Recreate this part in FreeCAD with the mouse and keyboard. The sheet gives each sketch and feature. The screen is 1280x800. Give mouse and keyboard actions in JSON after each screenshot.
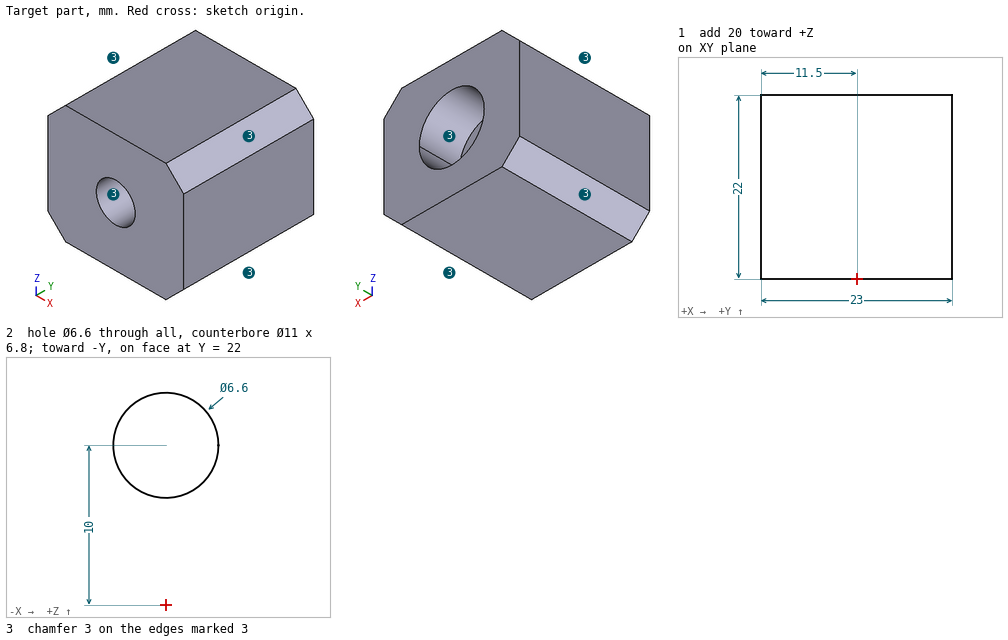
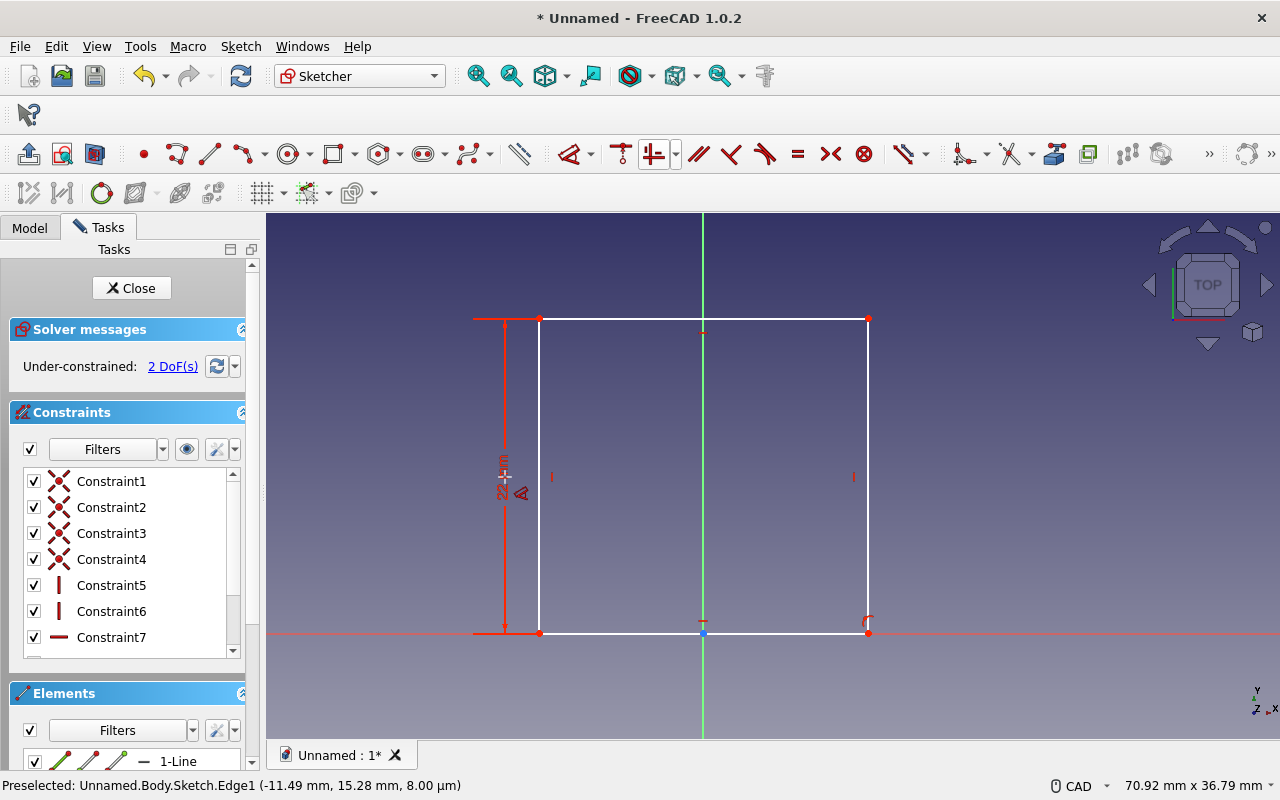
{"action": "left_click", "coordinate": [638, 634]}
{"action": "left_click", "coordinate": [628, 668]}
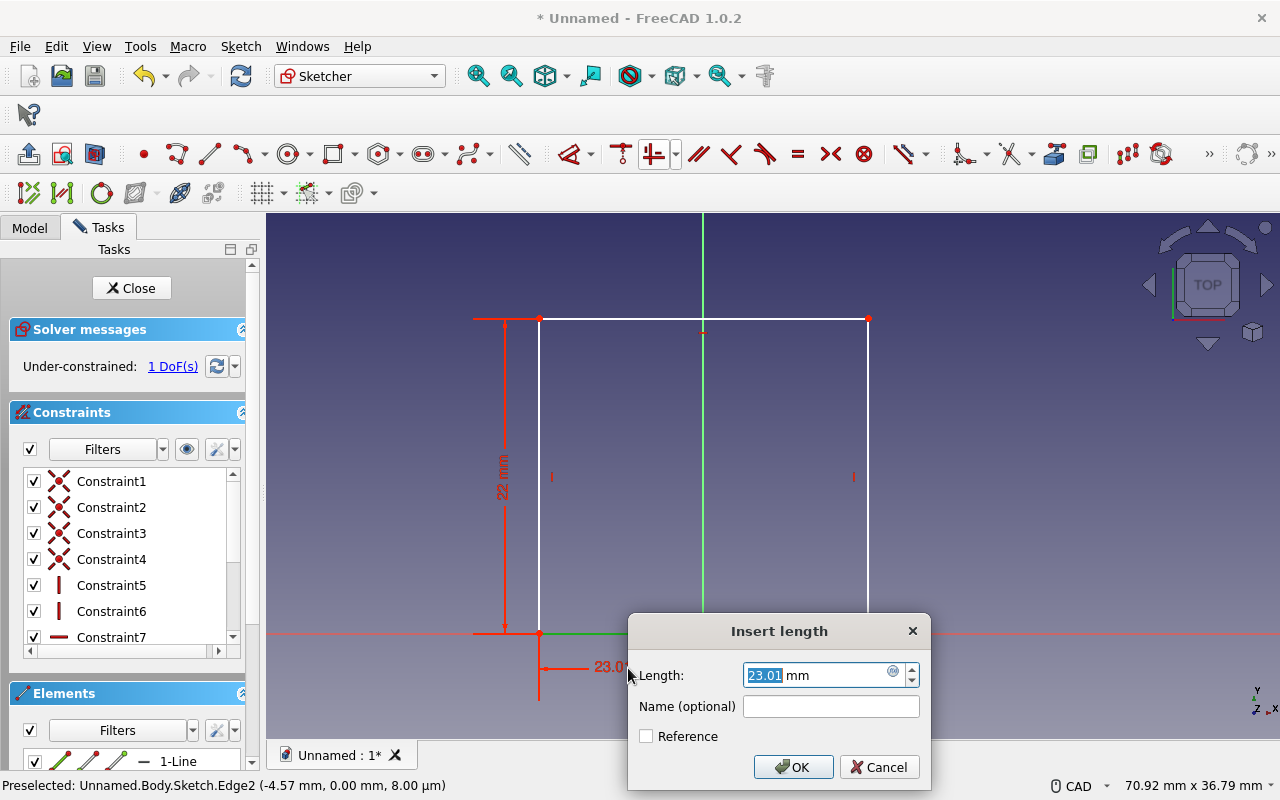
{"action": "type", "text": "23"}
{"action": "key", "text": "Return"}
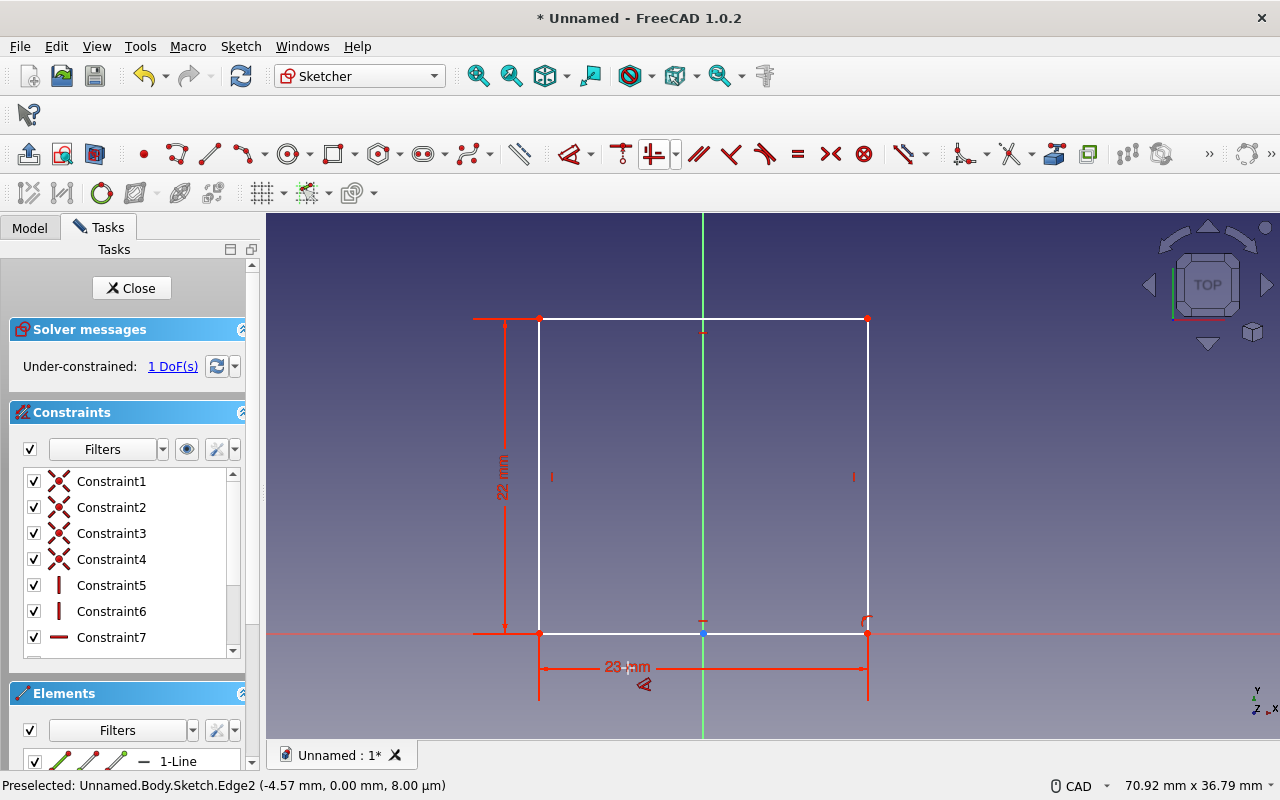
{"action": "left_click", "coordinate": [539, 319]}
{"action": "left_click", "coordinate": [621, 285]}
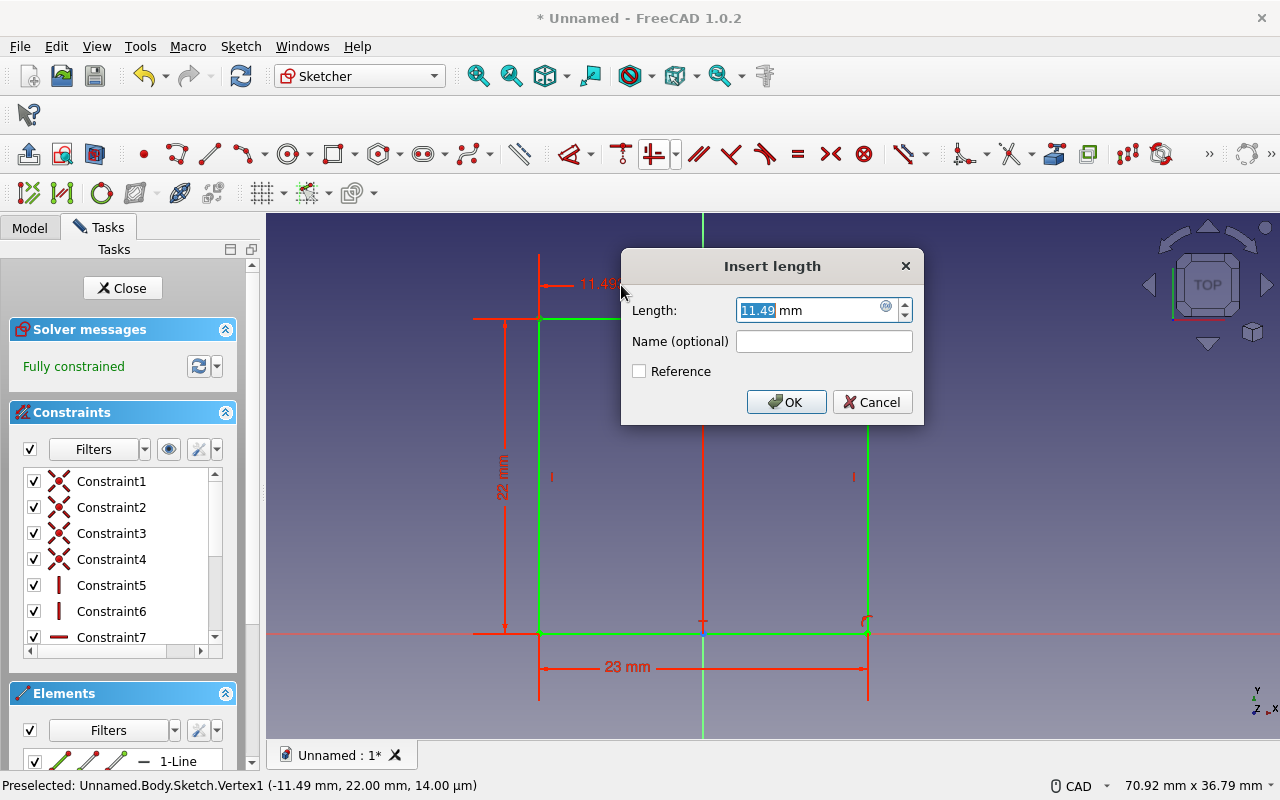
{"action": "type", "text": "11.5"}
{"action": "key", "text": "Return"}
{"action": "key", "text": "Escape"}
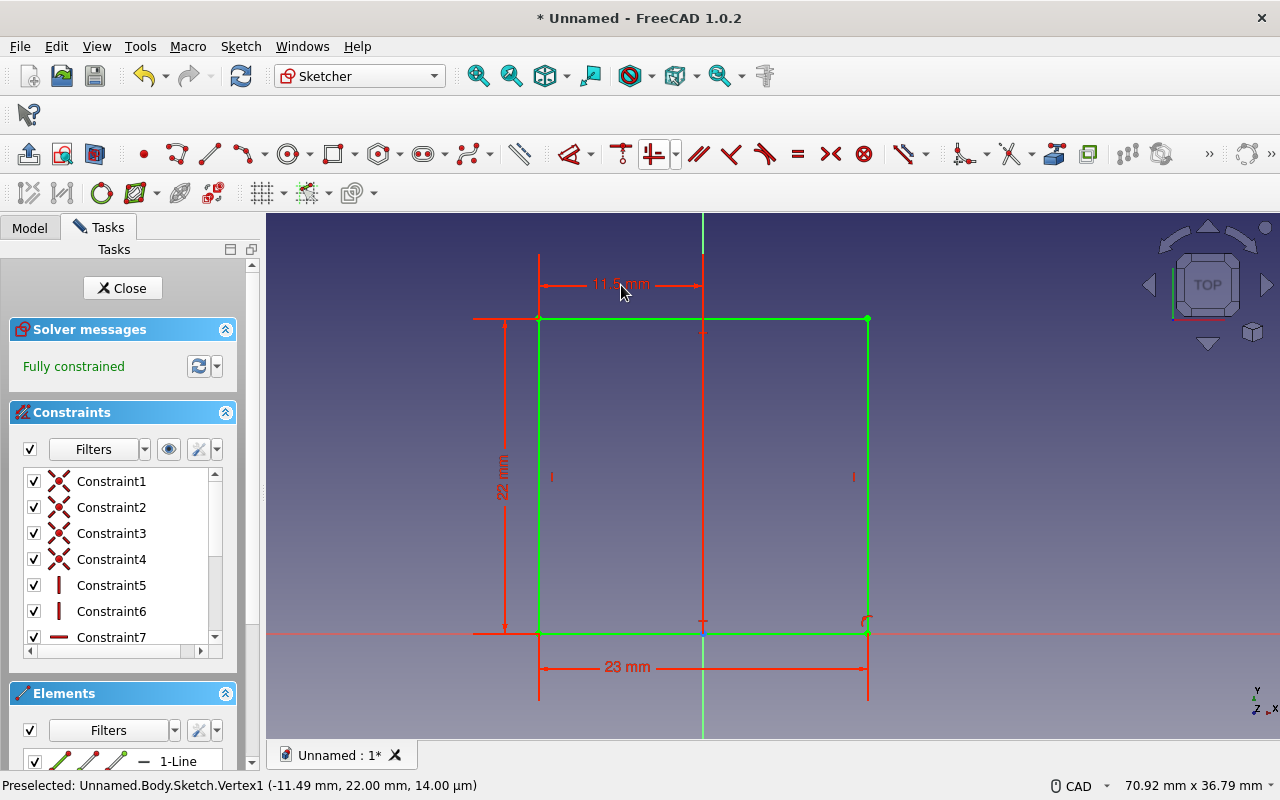
{"action": "left_click", "coordinate": [123, 288]}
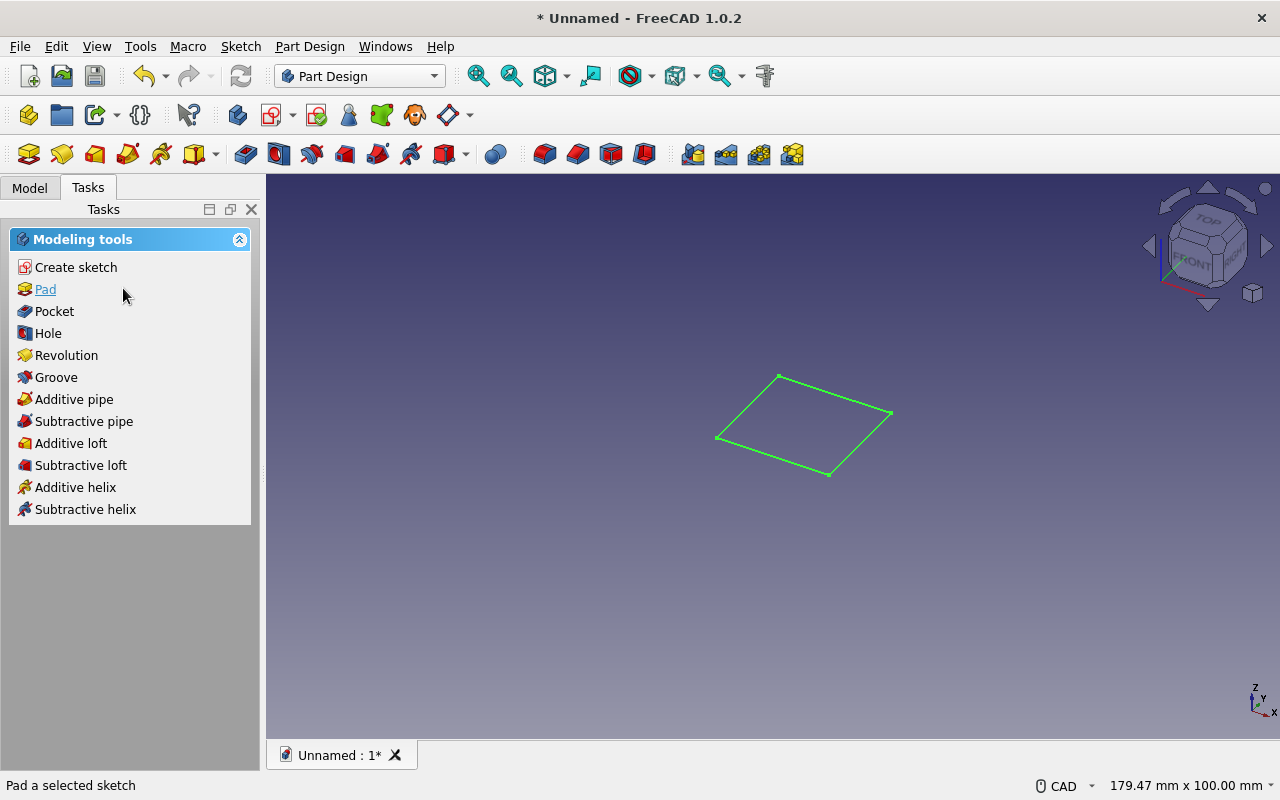
{"action": "left_click", "coordinate": [29, 154]}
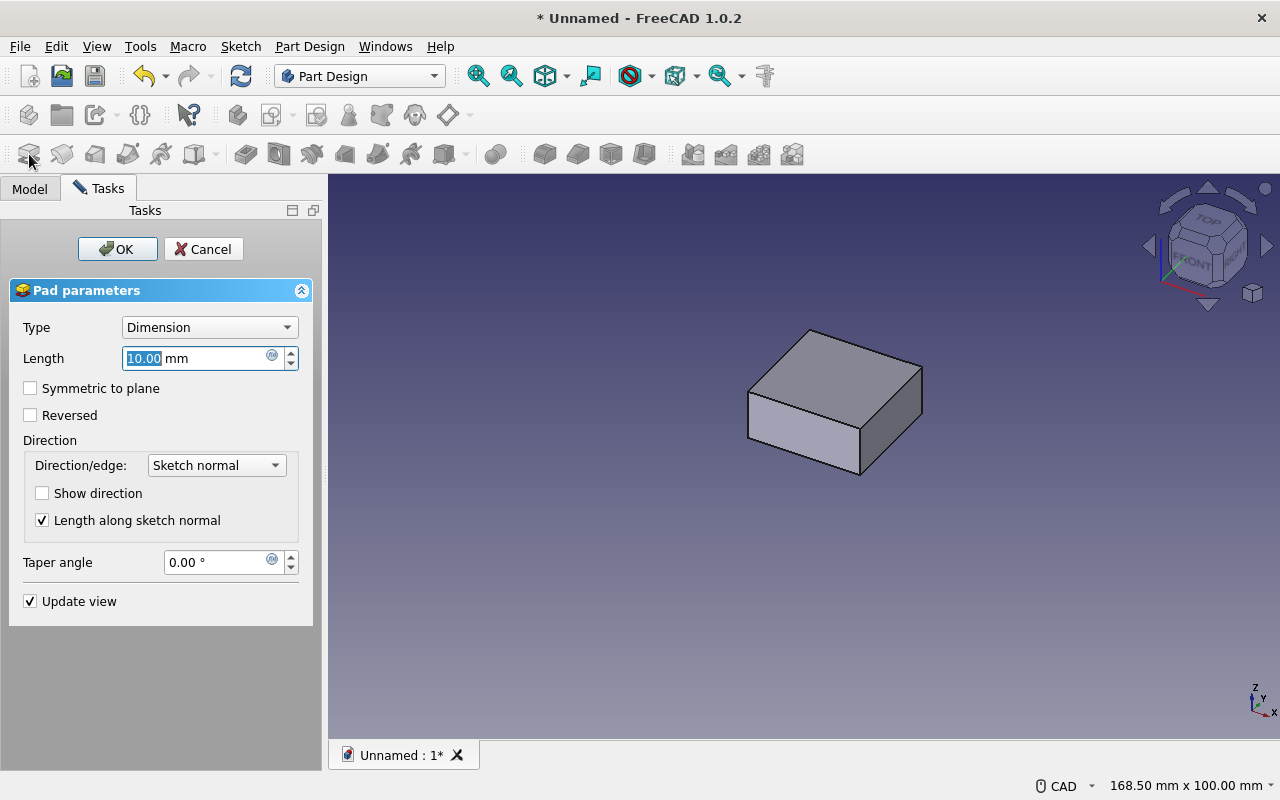
{"action": "type", "text": "20"}
{"action": "key", "text": "Tab"}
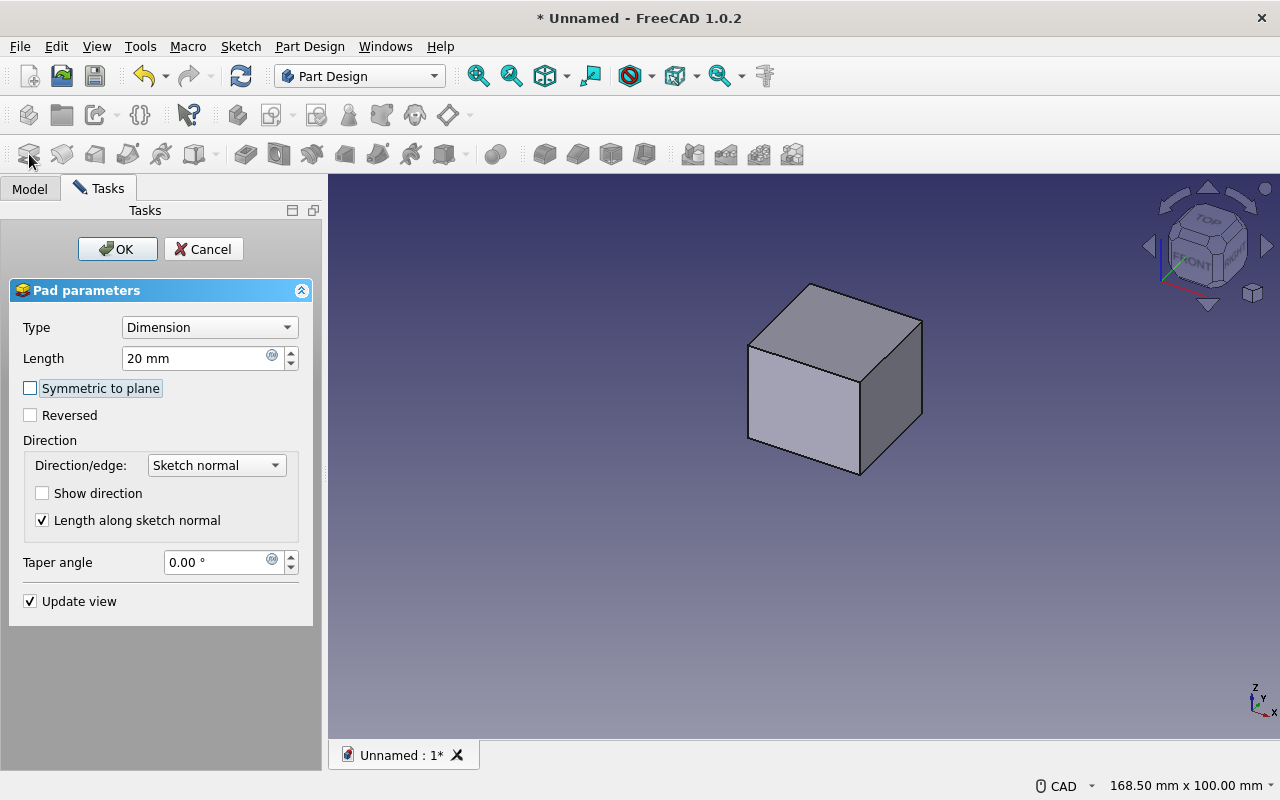
{"action": "left_click", "coordinate": [118, 249]}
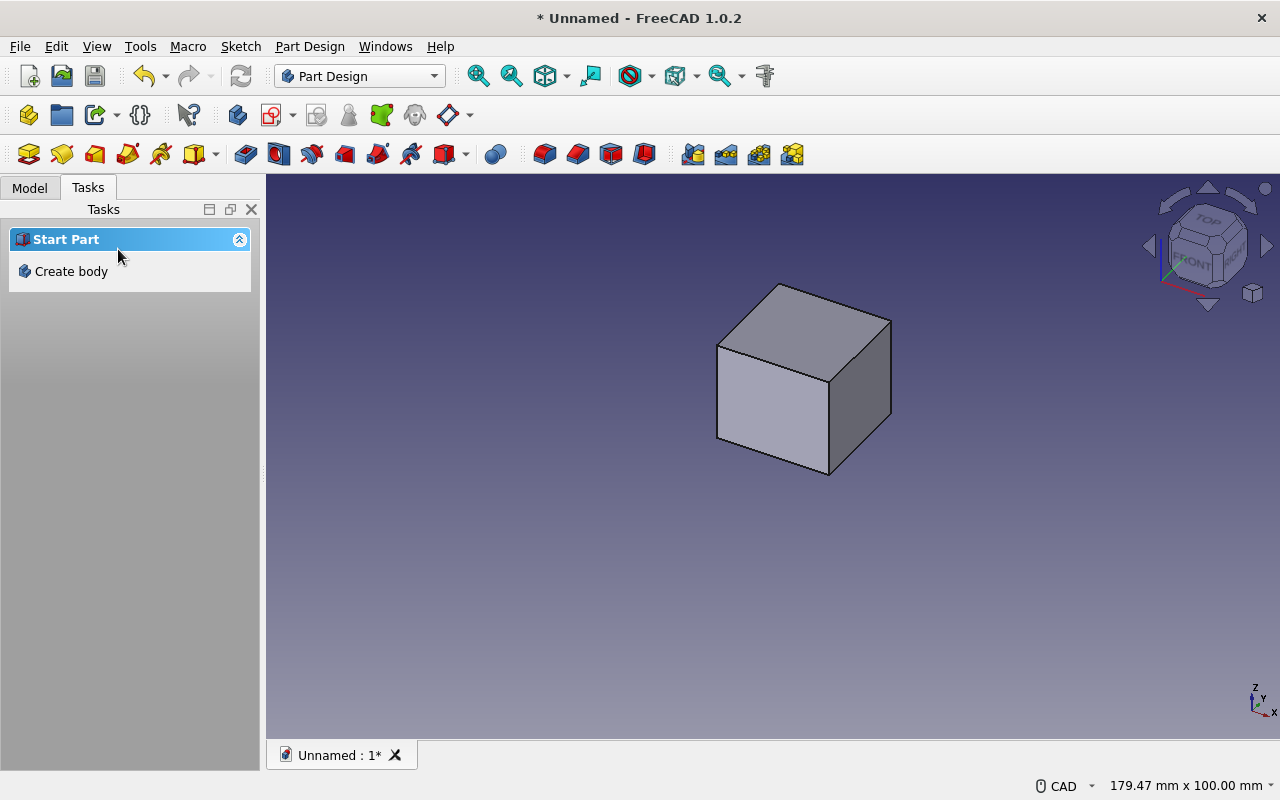
{"action": "left_click", "coordinate": [479, 76]}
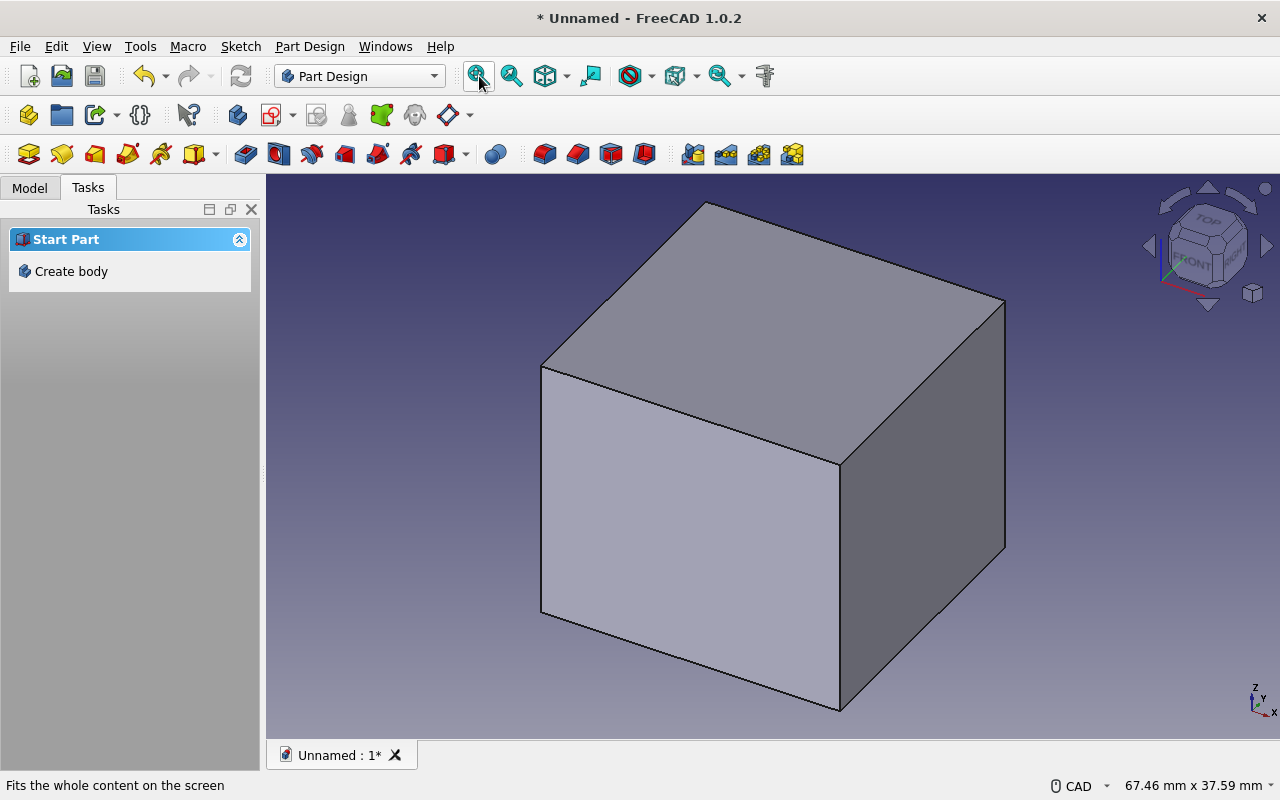
{"action": "key", "text": "4"}